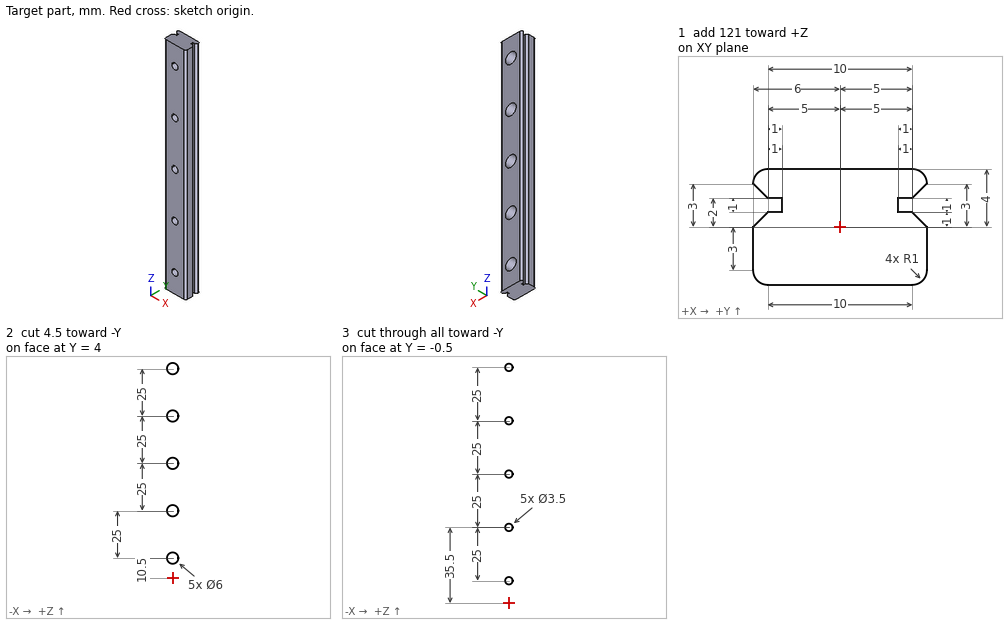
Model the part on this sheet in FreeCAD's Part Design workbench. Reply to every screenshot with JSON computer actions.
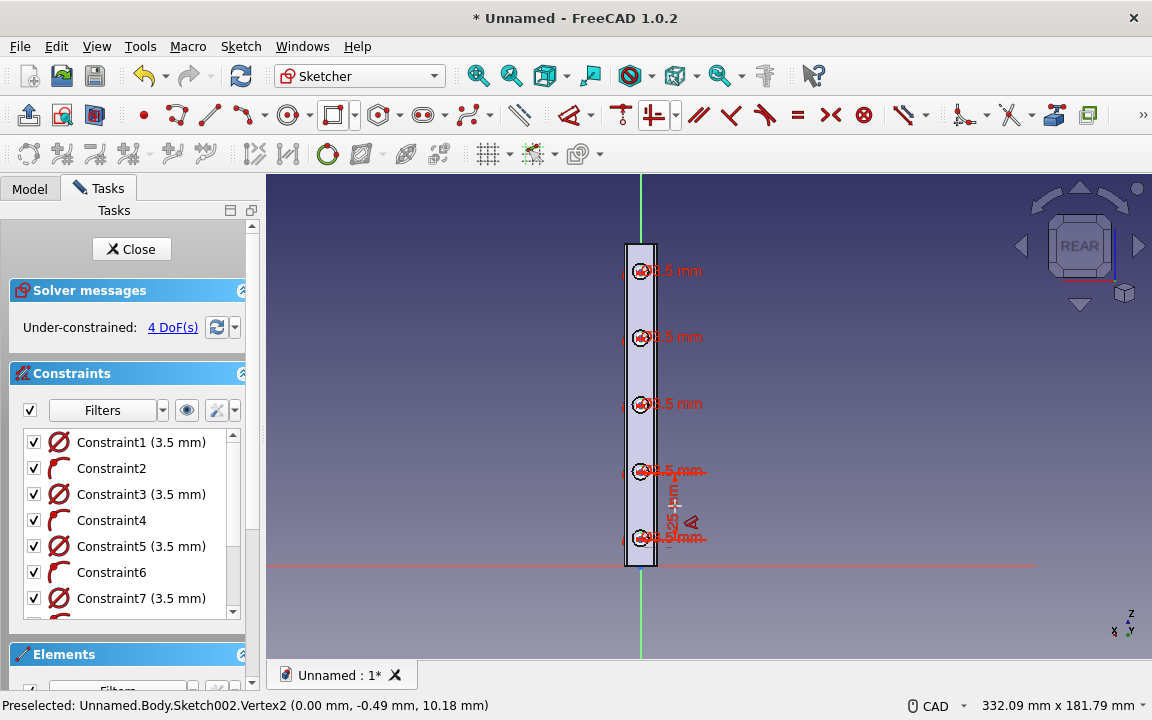
{"action": "left_click", "coordinate": [641, 473]}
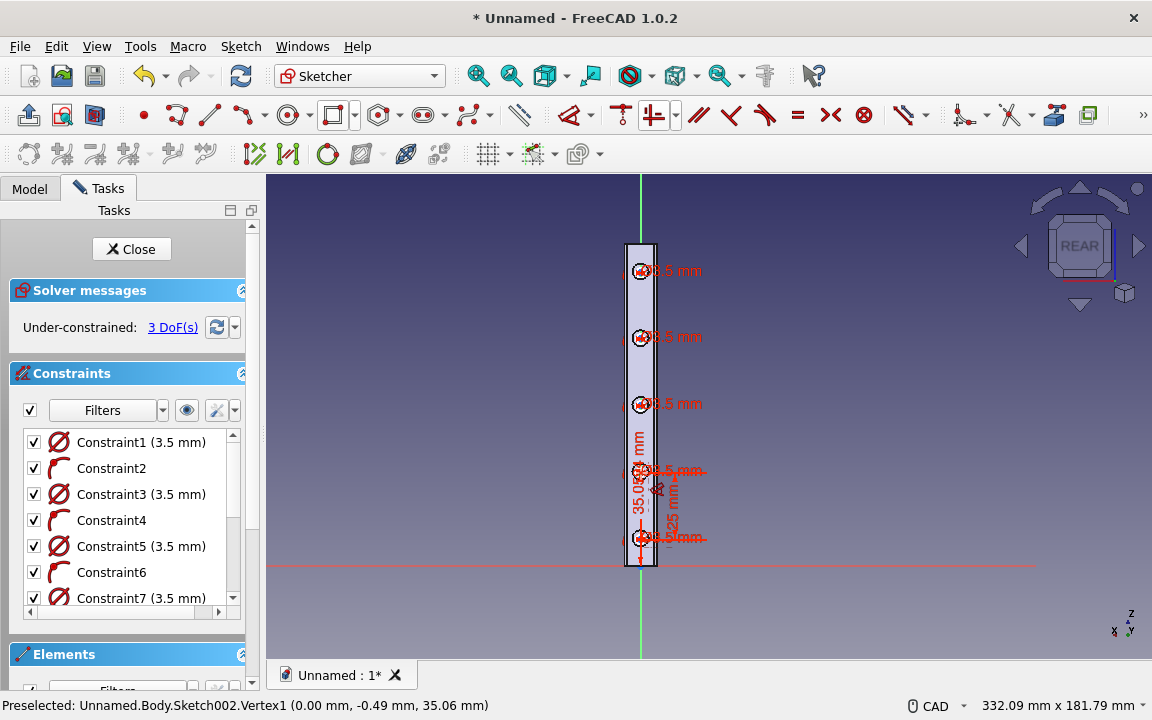
{"action": "left_click", "coordinate": [641, 406]}
{"action": "left_click", "coordinate": [675, 439]}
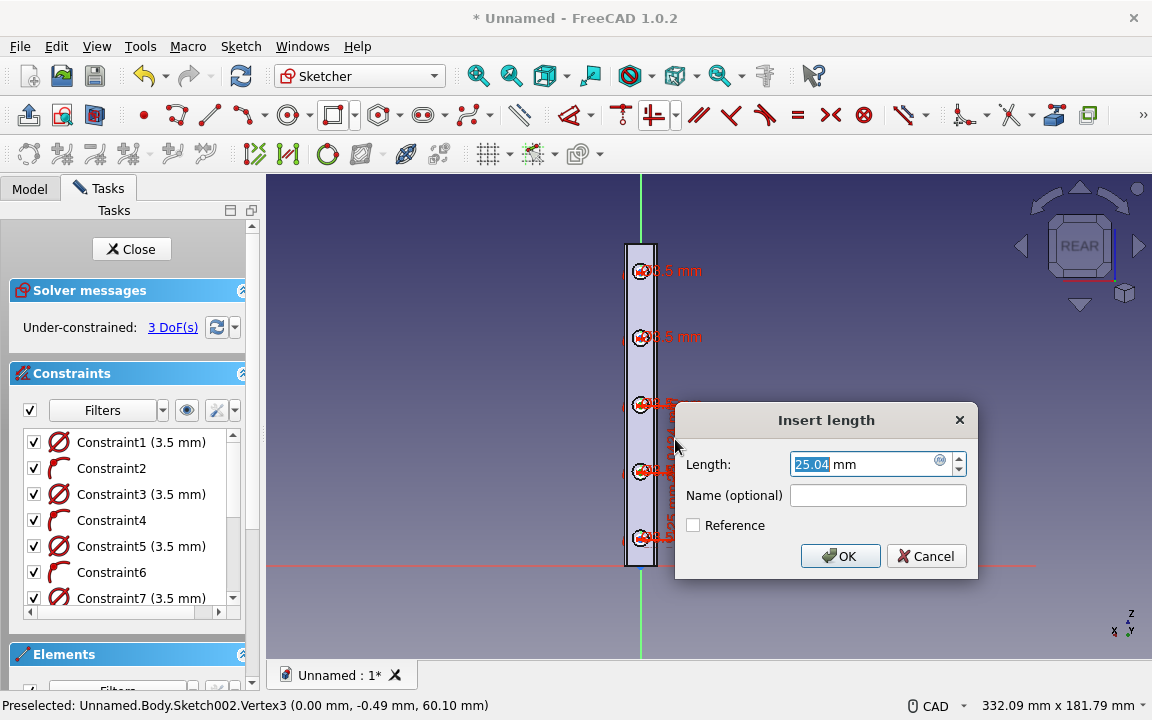
{"action": "type", "text": "25"}
{"action": "key", "text": "Return"}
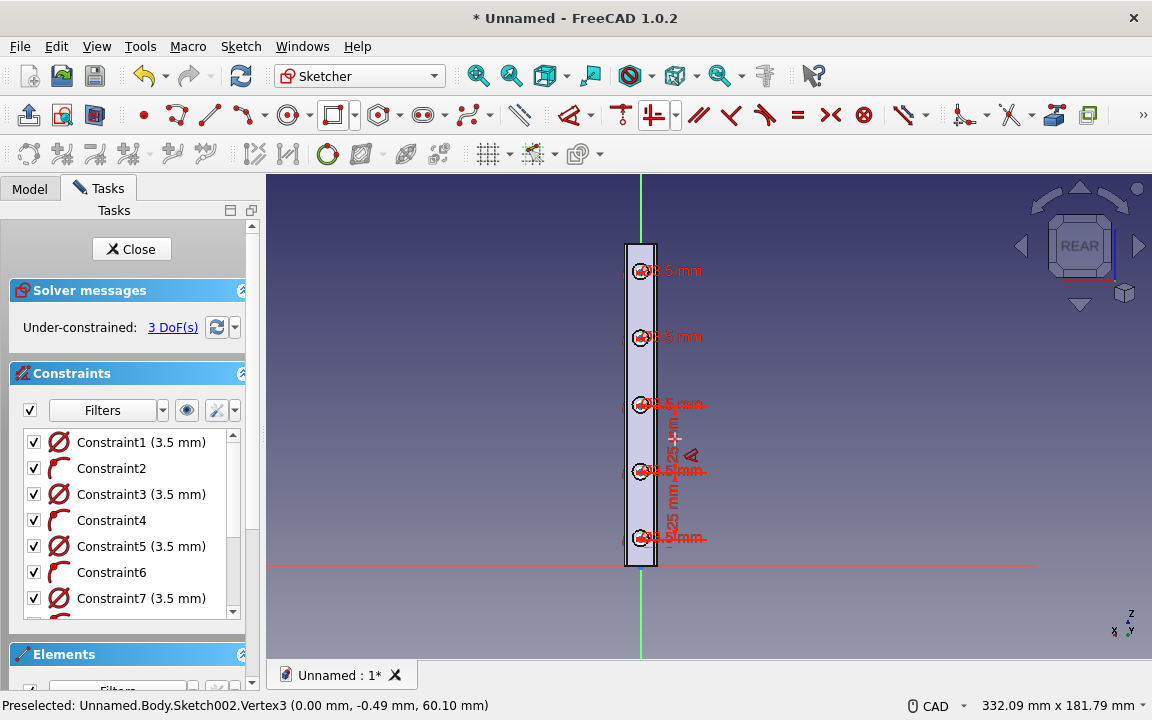
{"action": "left_click", "coordinate": [641, 406]}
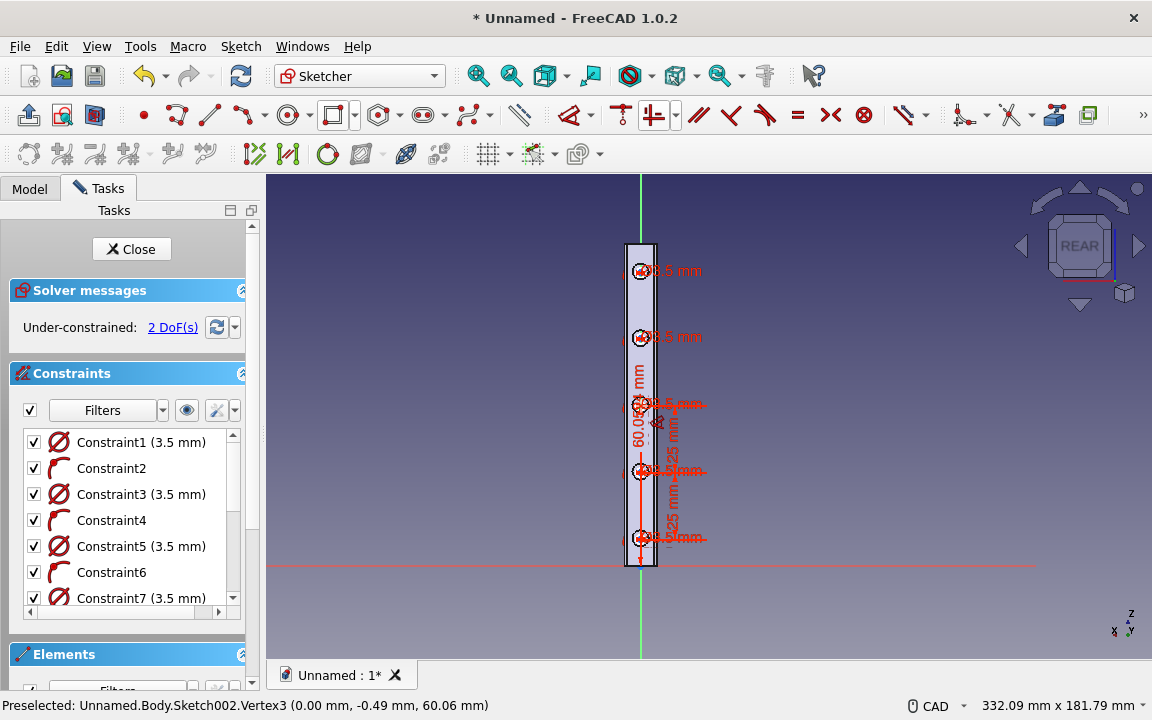
{"action": "left_click", "coordinate": [641, 339]}
{"action": "left_click", "coordinate": [675, 373]}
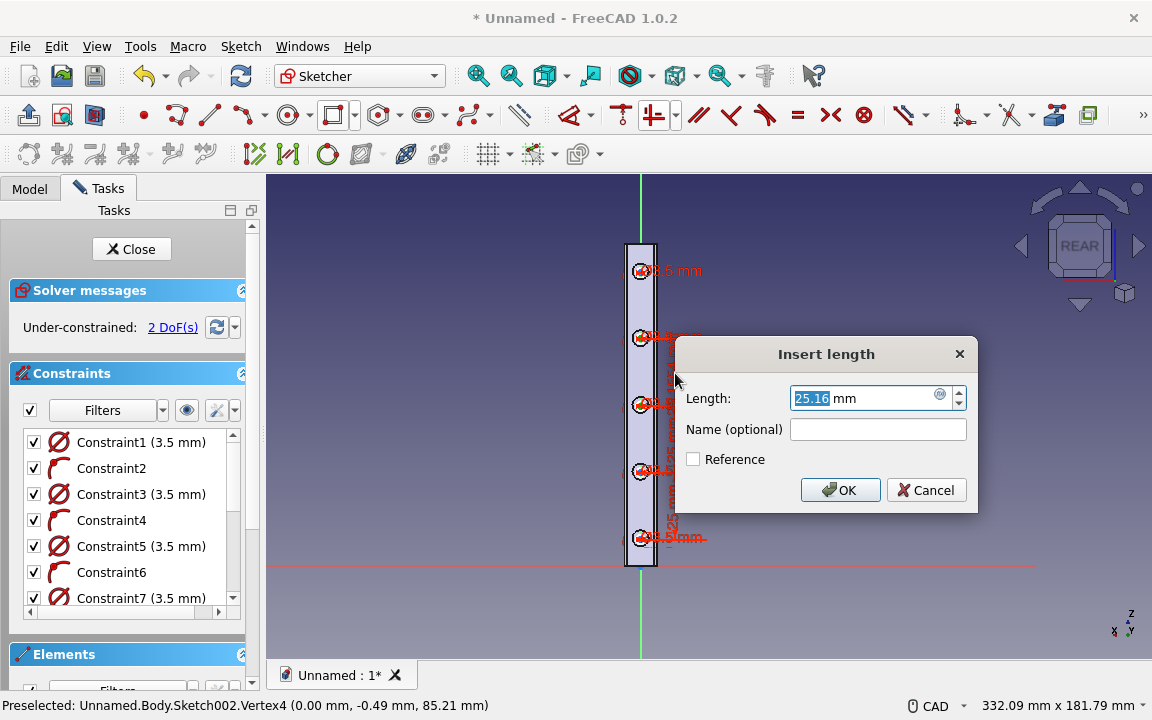
{"action": "type", "text": "25"}
{"action": "key", "text": "Return"}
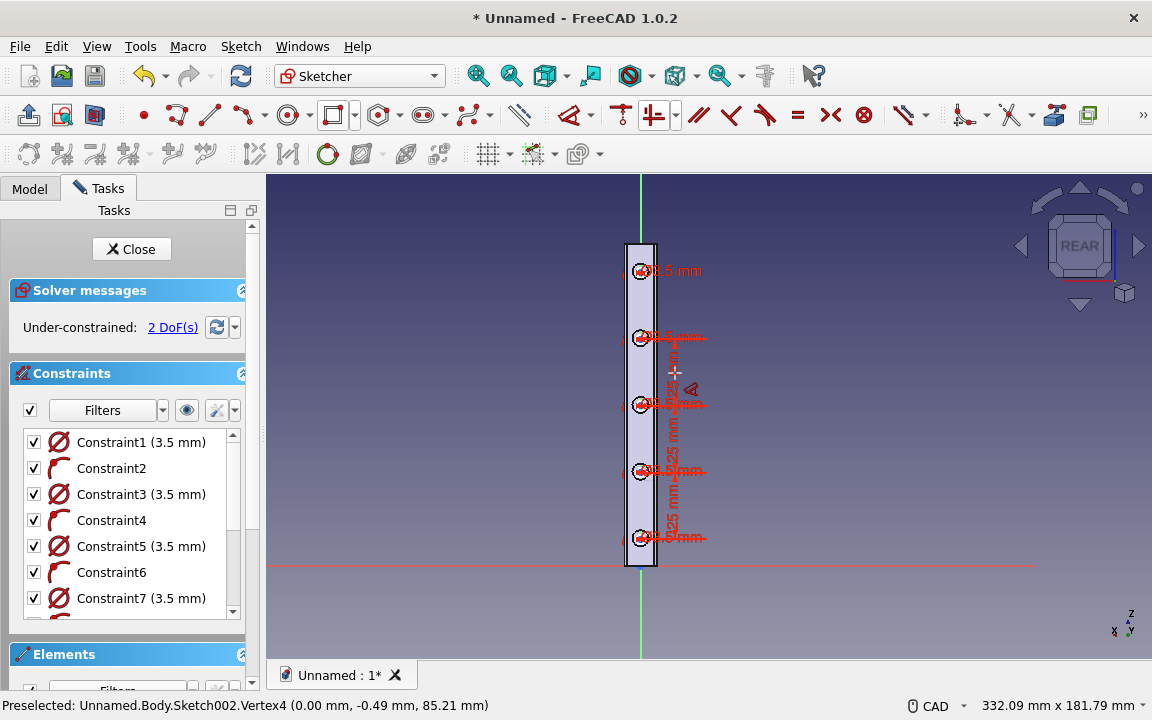
{"action": "left_click", "coordinate": [641, 339]}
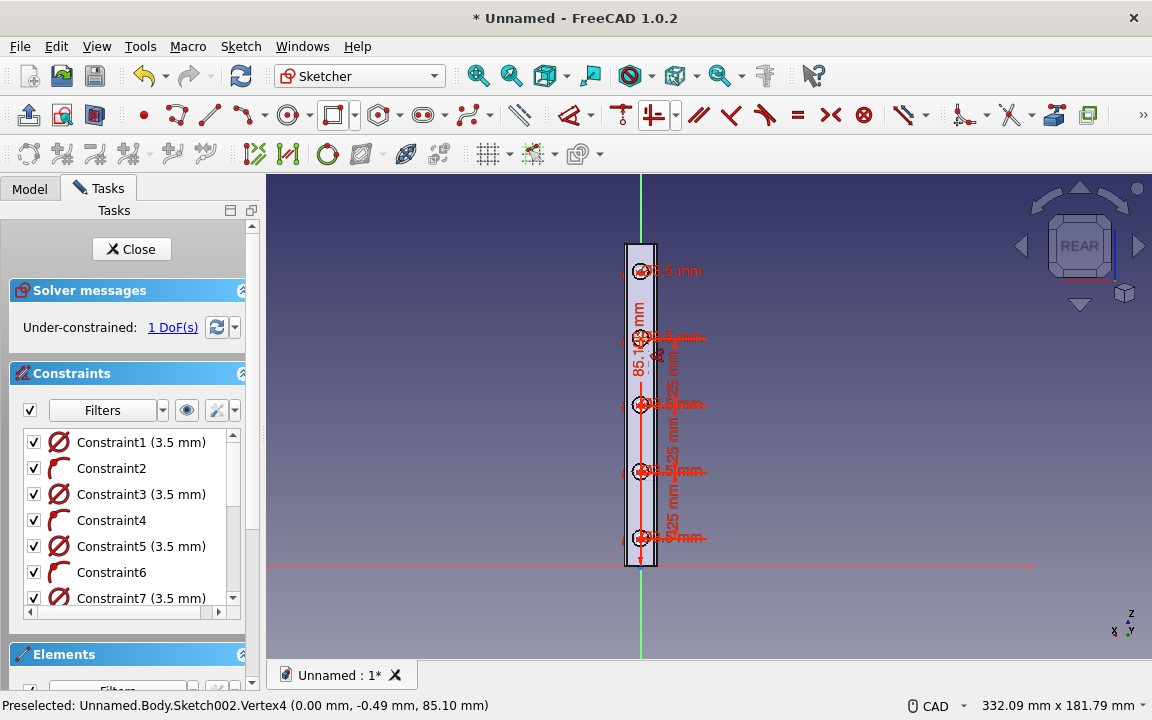
{"action": "left_click", "coordinate": [641, 273]}
{"action": "left_click", "coordinate": [675, 306]}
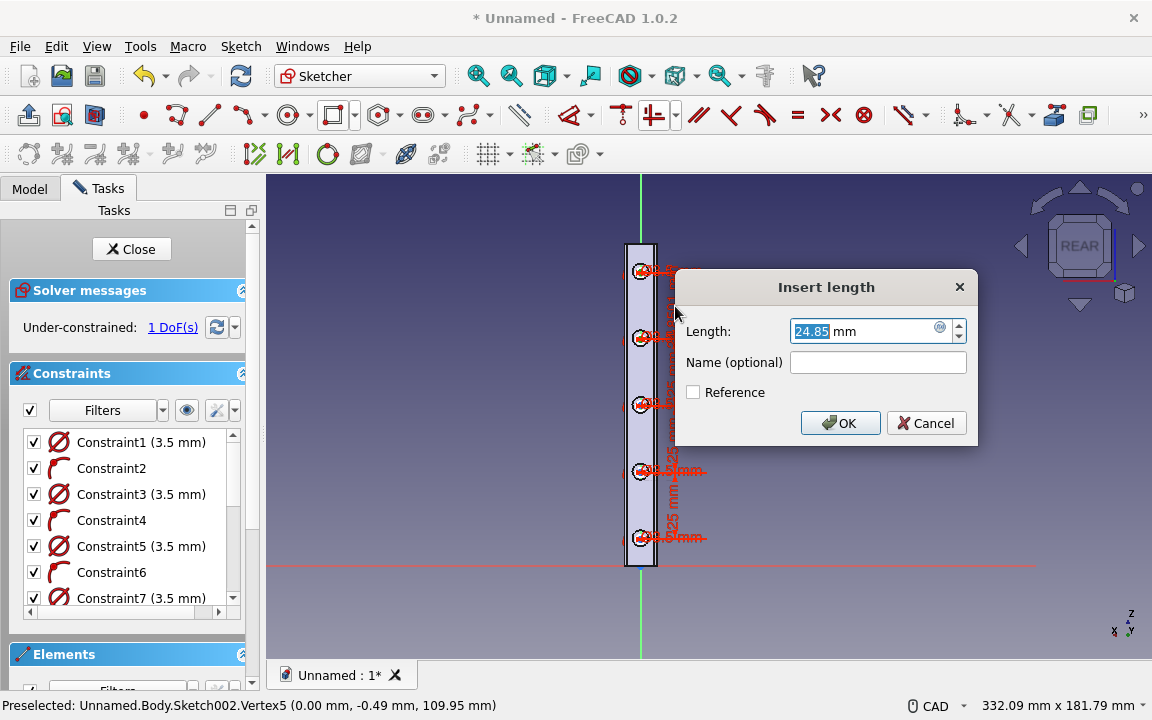
{"action": "type", "text": "25"}
{"action": "key", "text": "Return"}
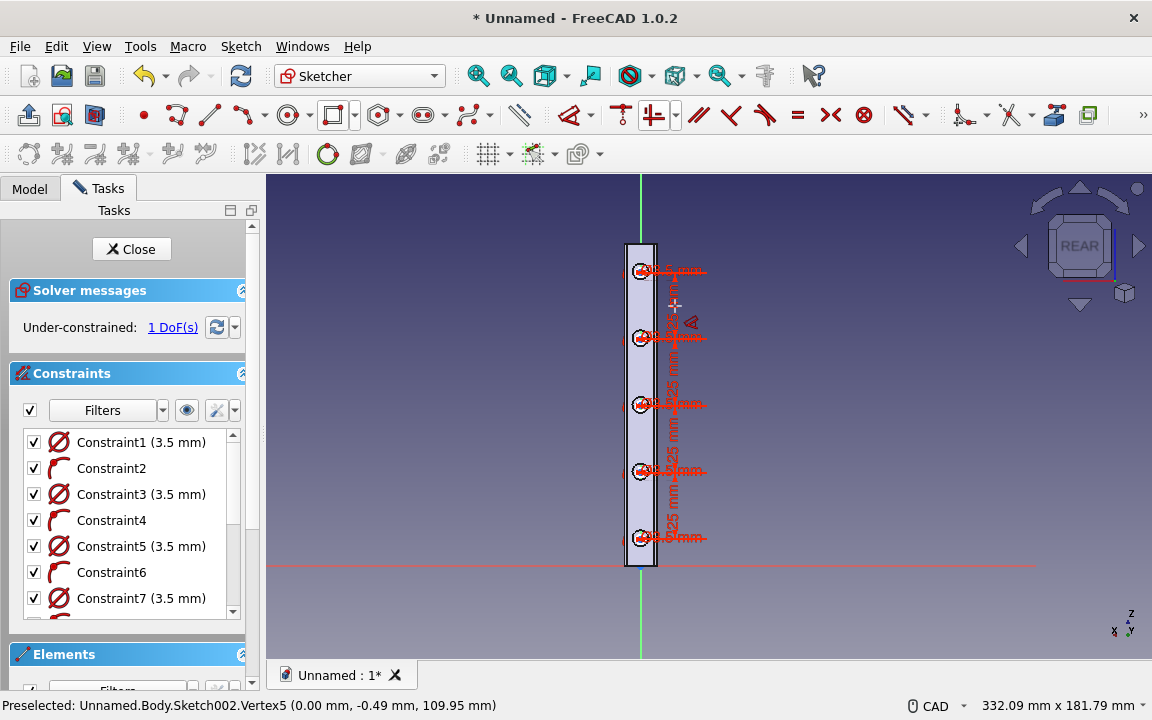
{"action": "left_click", "coordinate": [641, 473]}
{"action": "left_click", "coordinate": [675, 541]}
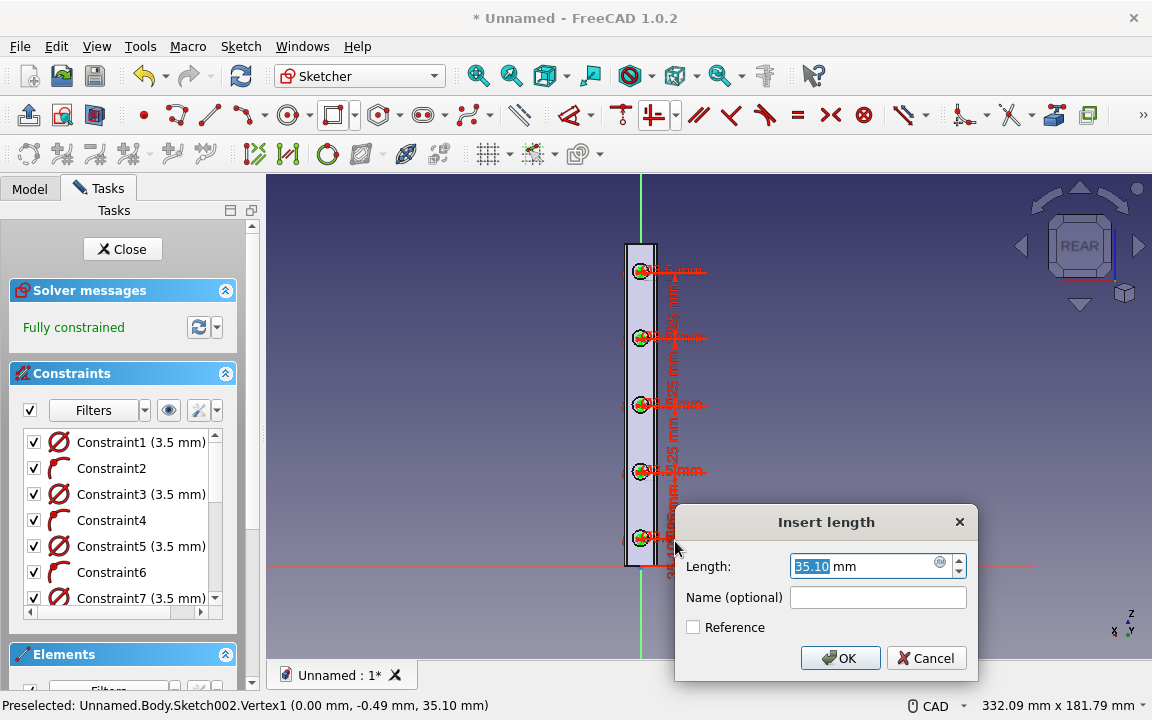
{"action": "type", "text": "35.5"}
{"action": "key", "text": "Return"}
{"action": "key", "text": "Escape"}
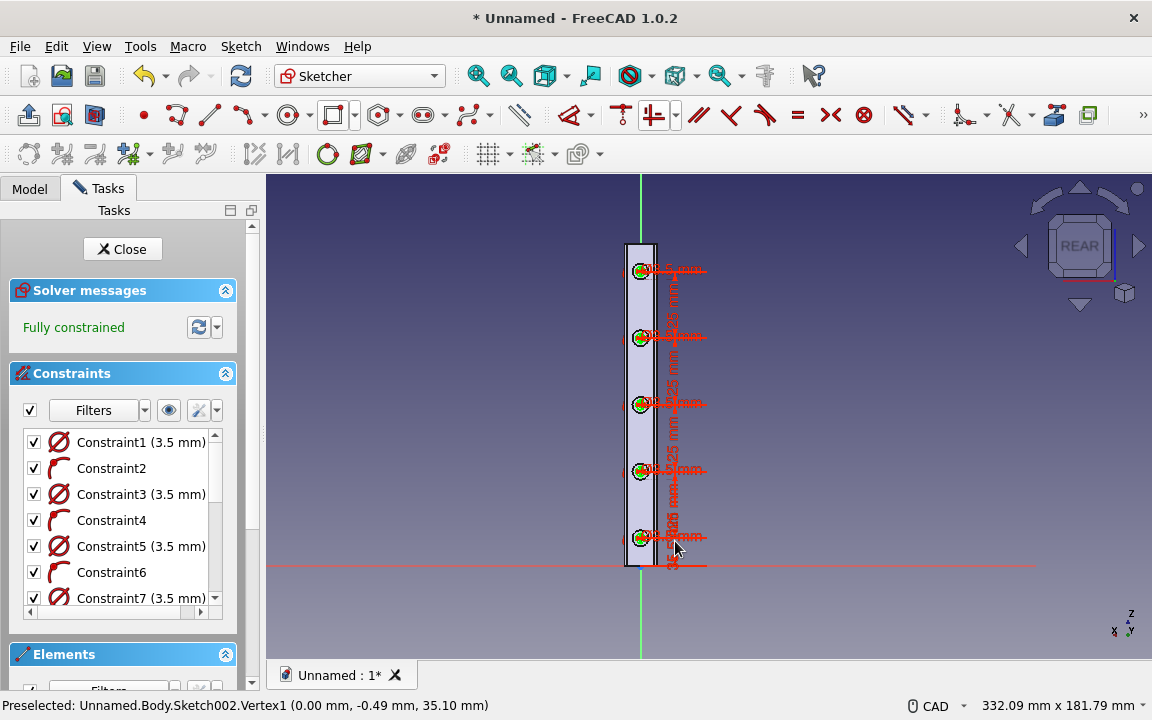
{"action": "left_click", "coordinate": [123, 249]}